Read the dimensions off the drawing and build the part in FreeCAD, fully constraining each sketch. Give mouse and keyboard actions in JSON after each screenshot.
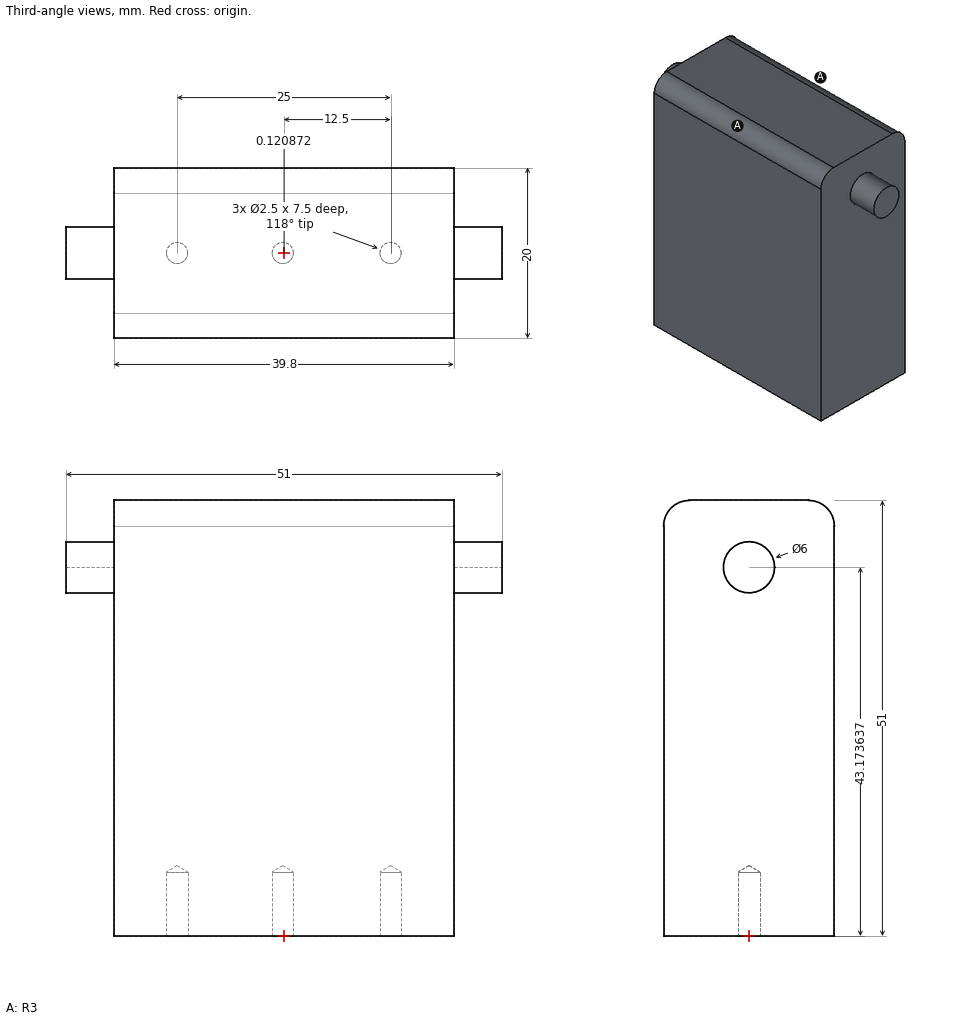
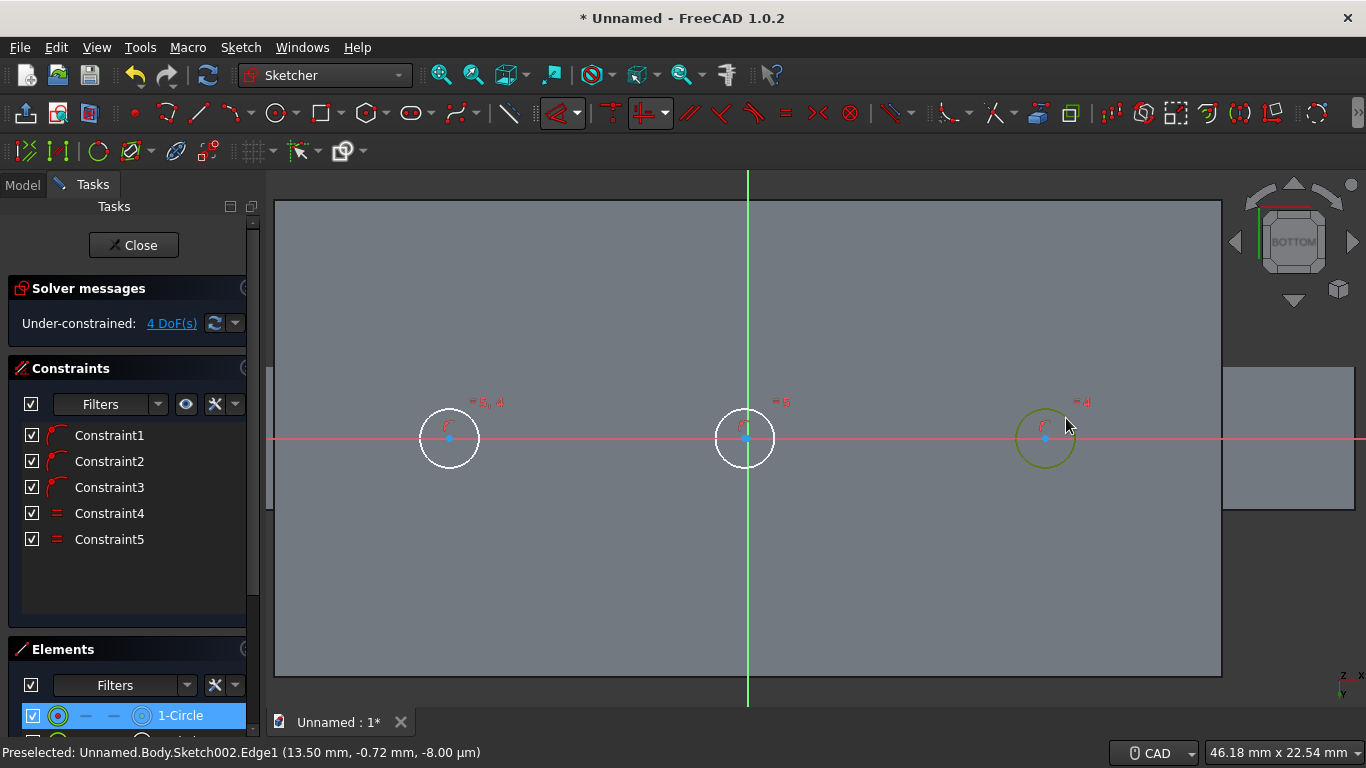
{"action": "left_click", "coordinate": [580, 114]}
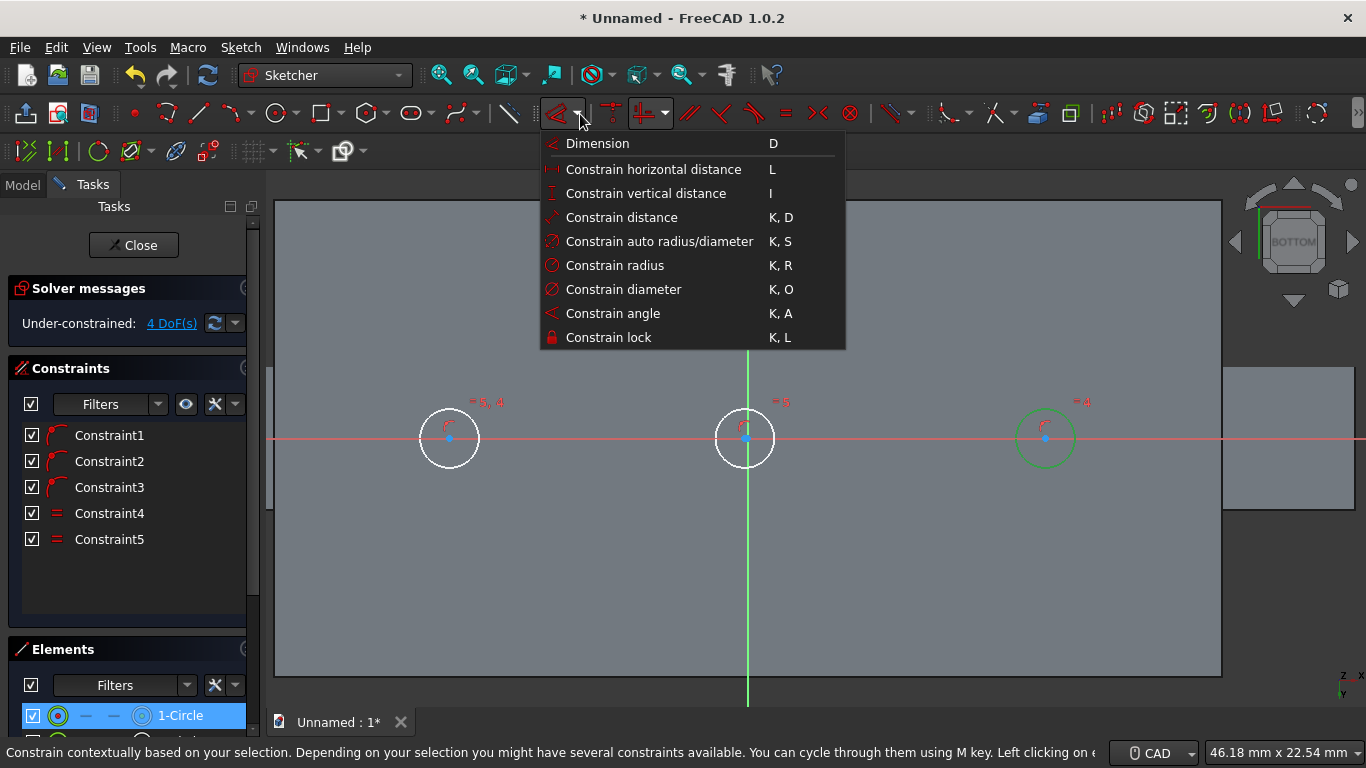
{"action": "left_click", "coordinate": [693, 289]}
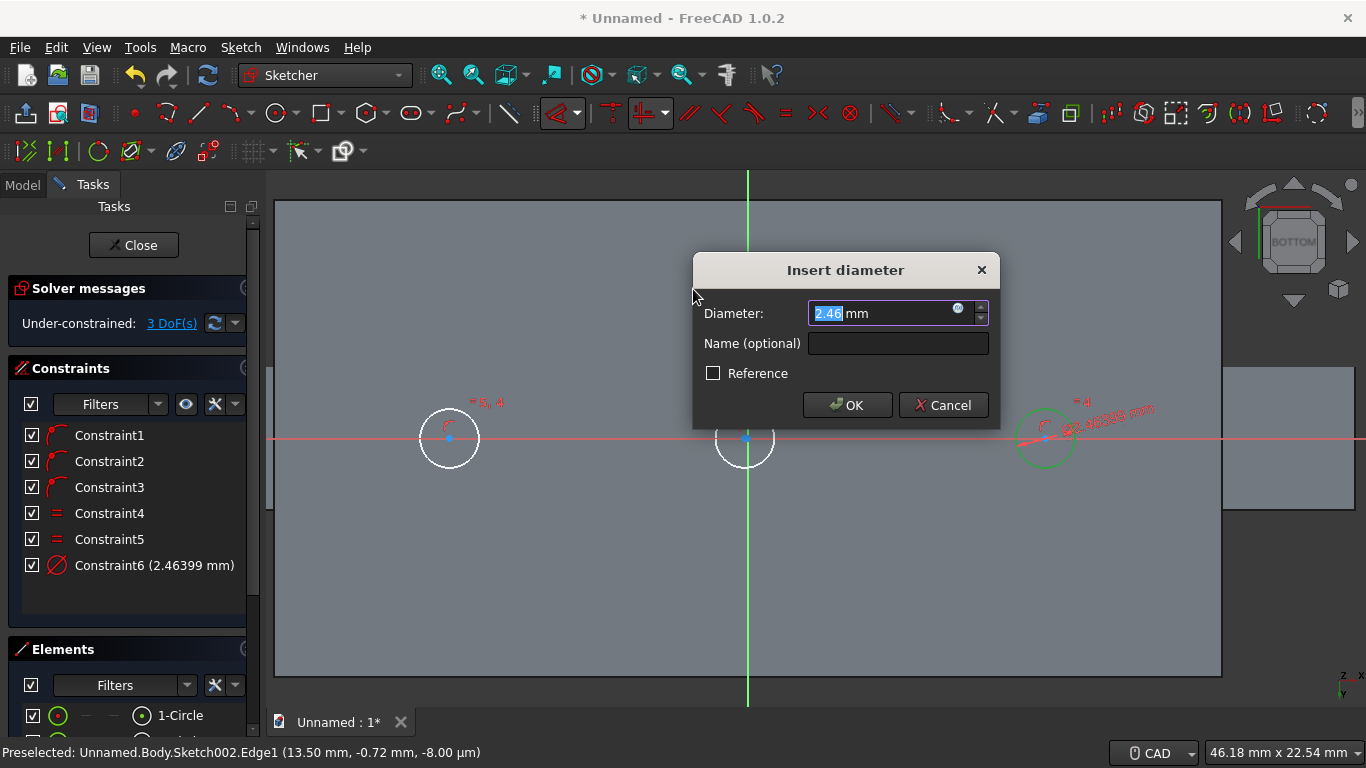
{"action": "type", "text": "2.5"}
{"action": "key", "text": "Return"}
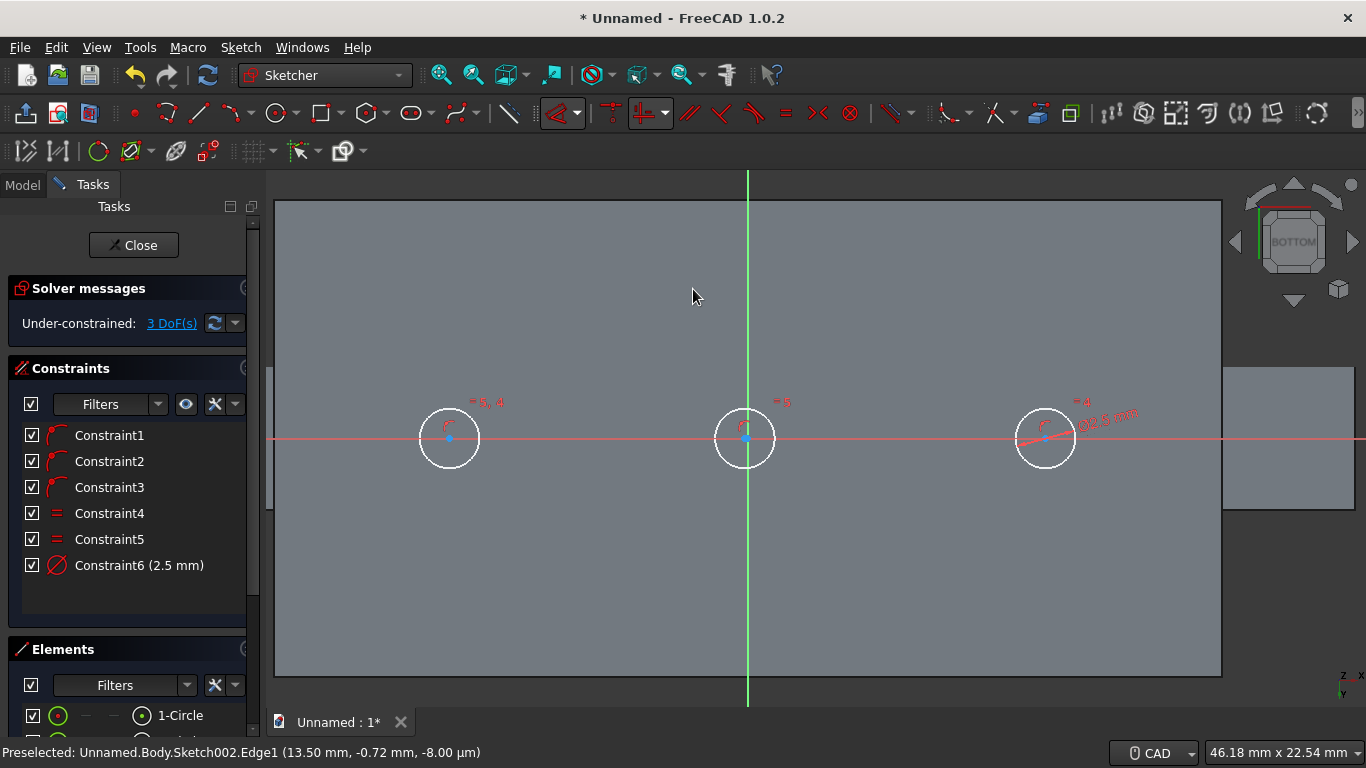
{"action": "left_click", "coordinate": [1046, 438]}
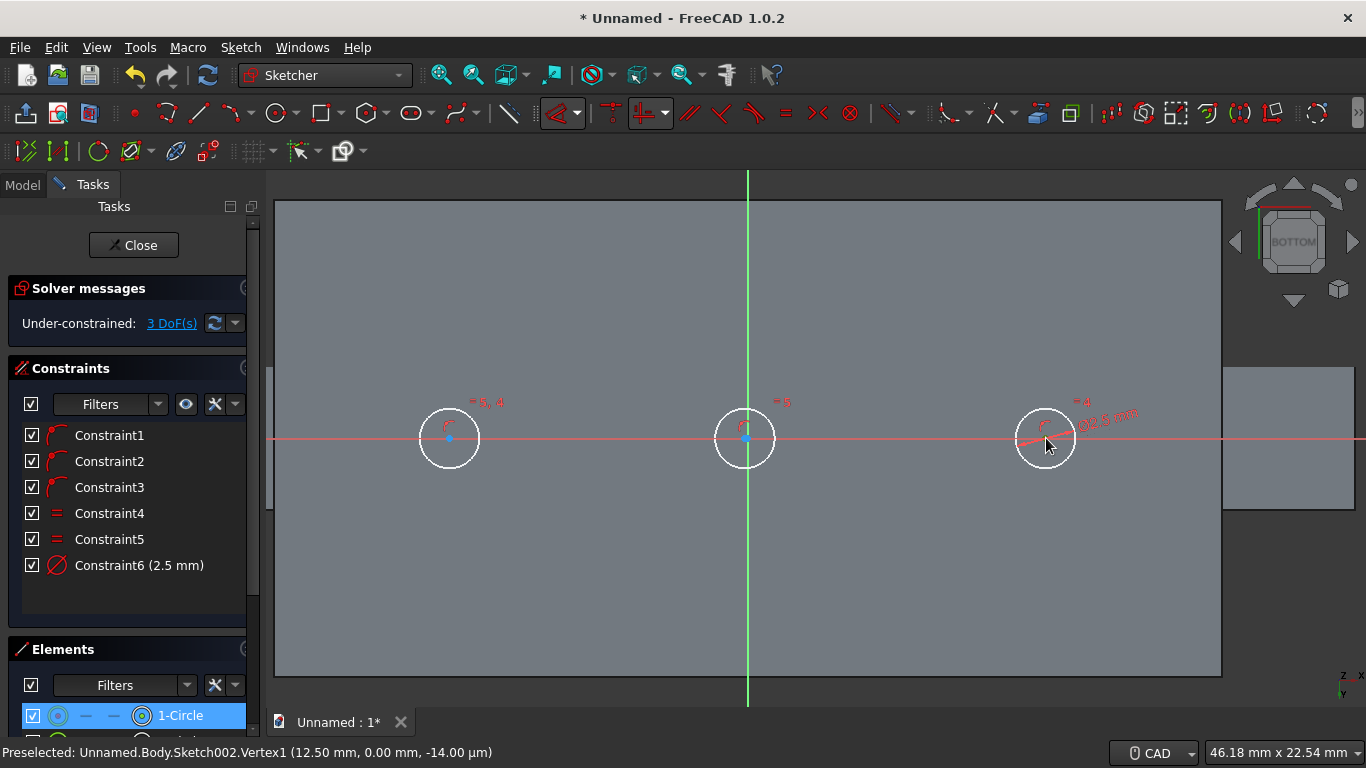
{"action": "left_click", "coordinate": [450, 438]}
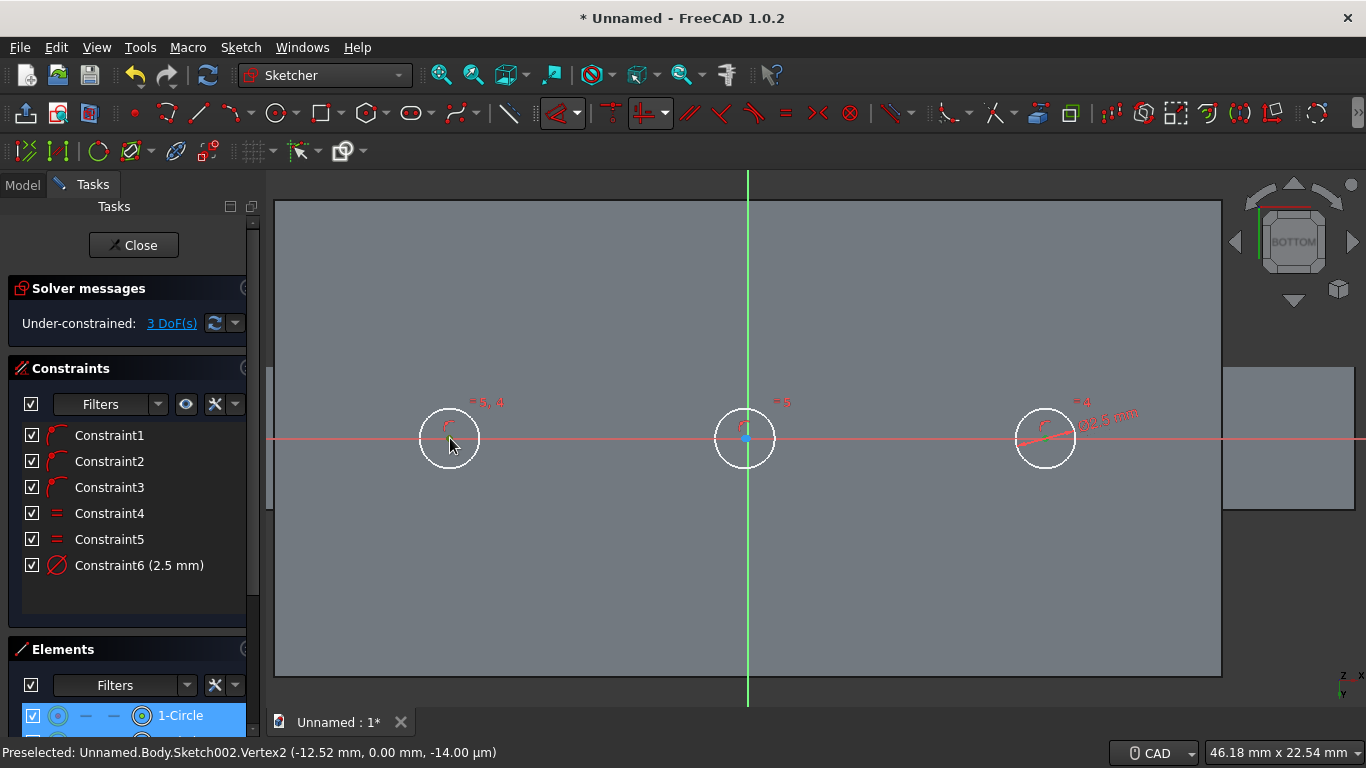
{"action": "key", "text": "l"}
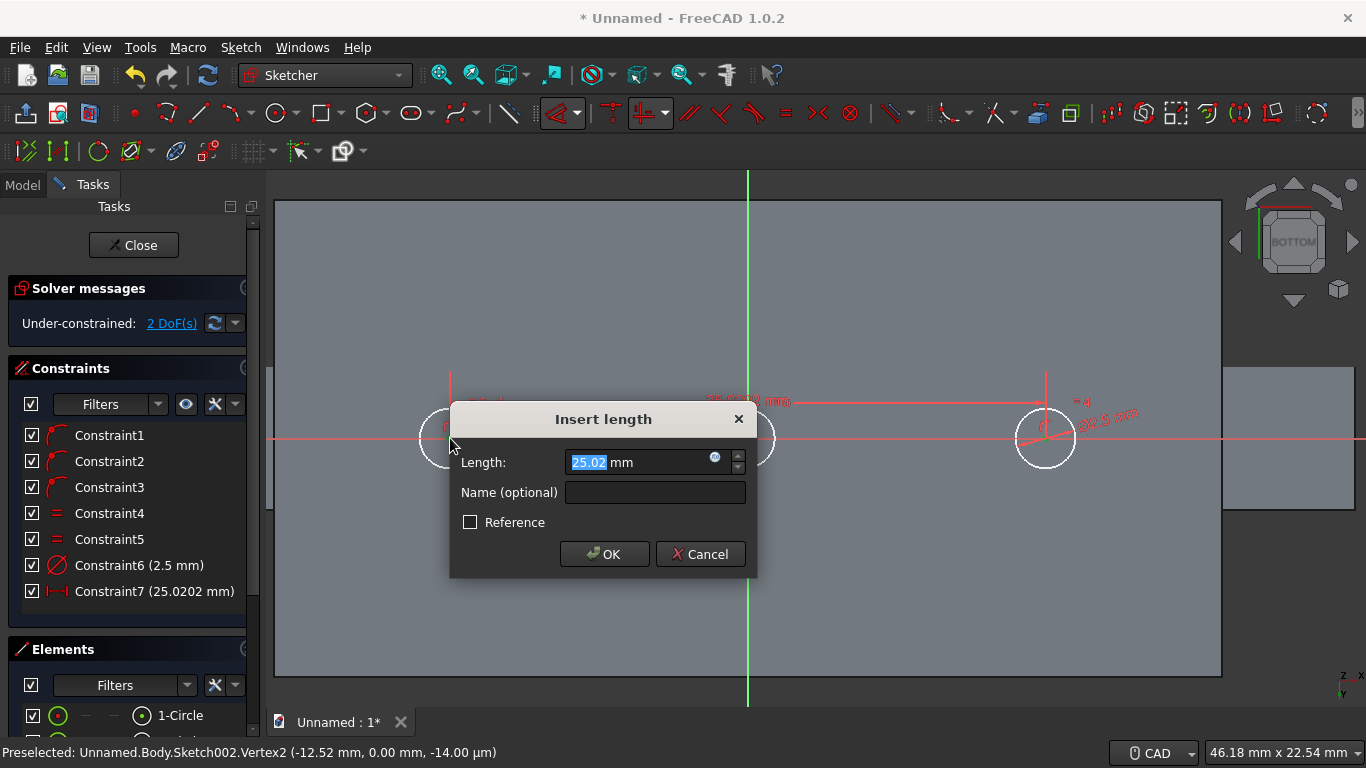
{"action": "type", "text": "25"}
{"action": "key", "text": "Return"}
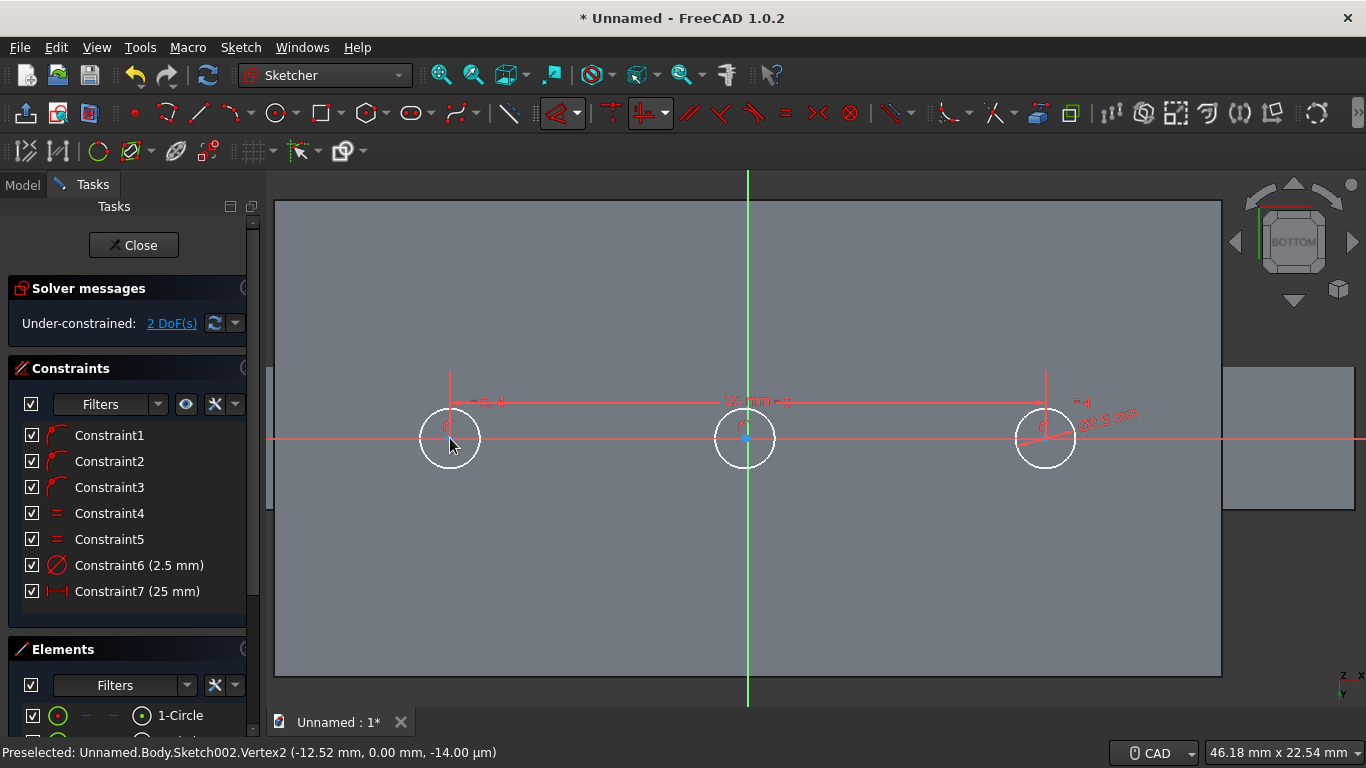
{"action": "left_click", "coordinate": [1046, 438]}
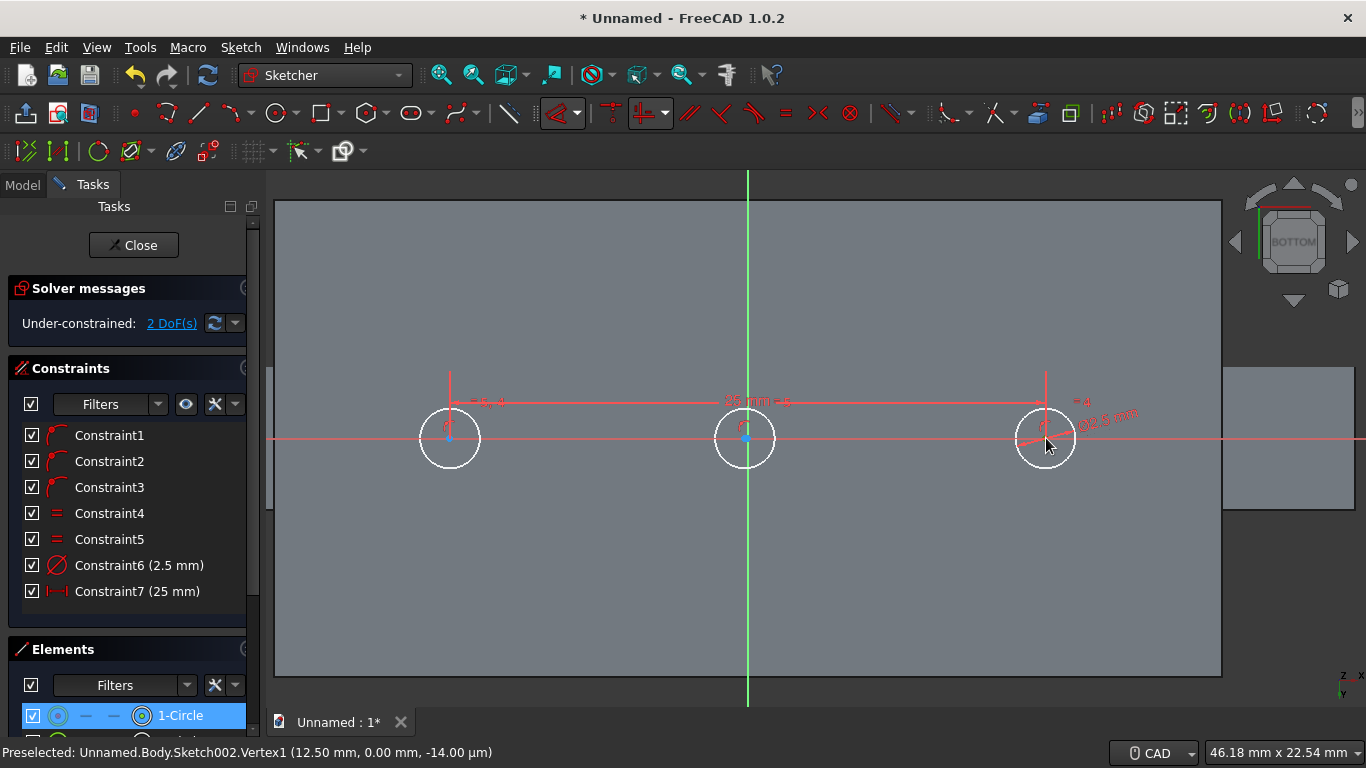
{"action": "key", "text": "l"}